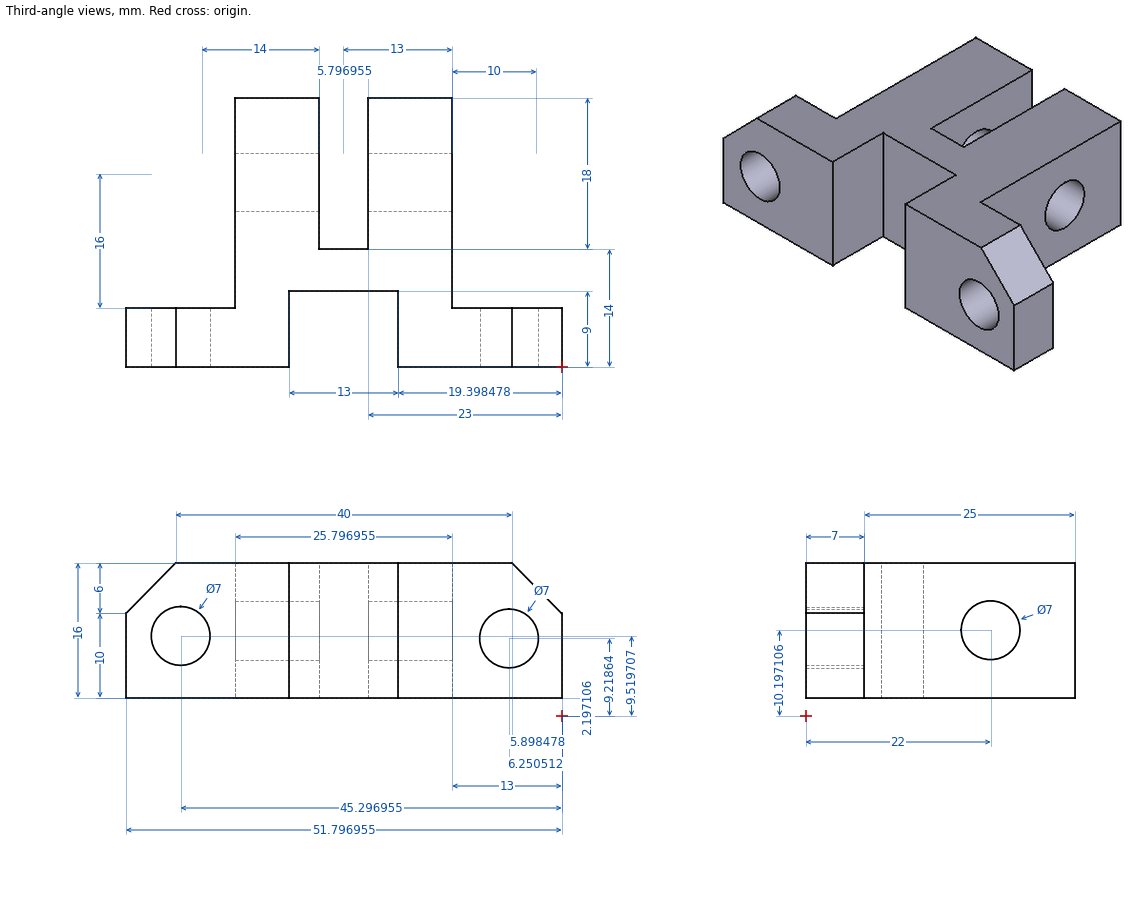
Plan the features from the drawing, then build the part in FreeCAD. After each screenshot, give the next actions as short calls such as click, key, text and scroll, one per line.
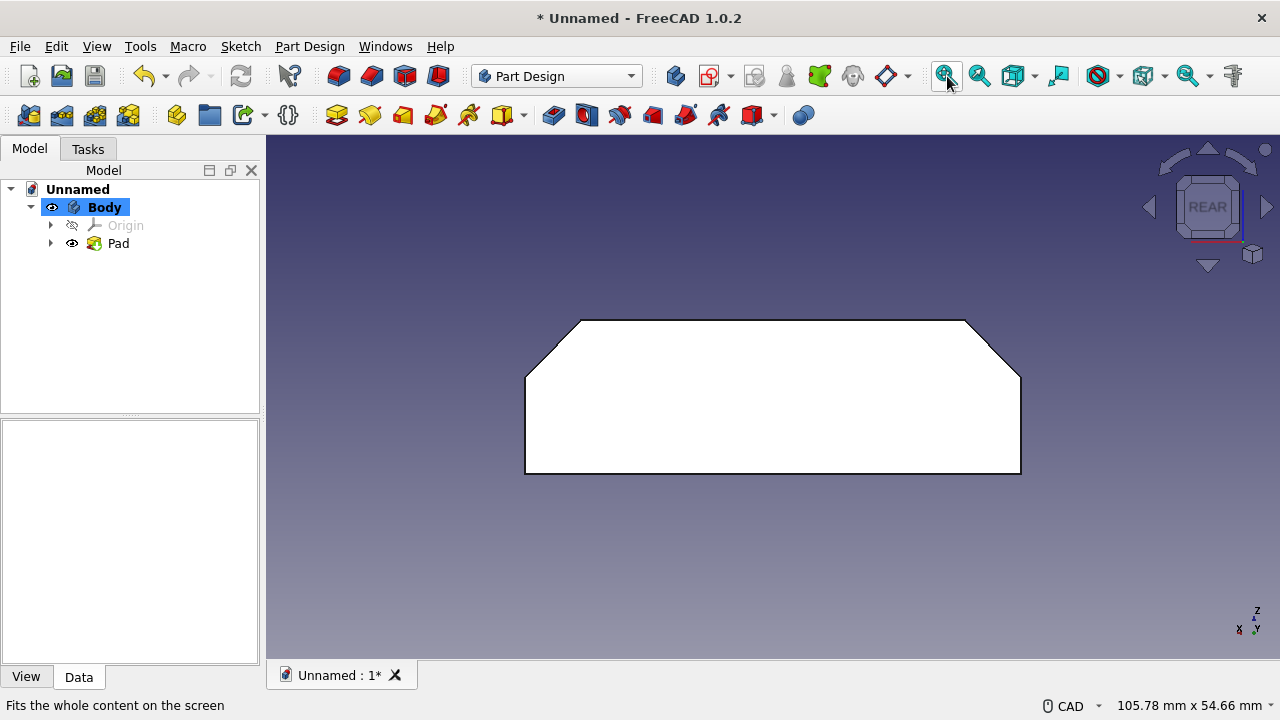
click(631, 396)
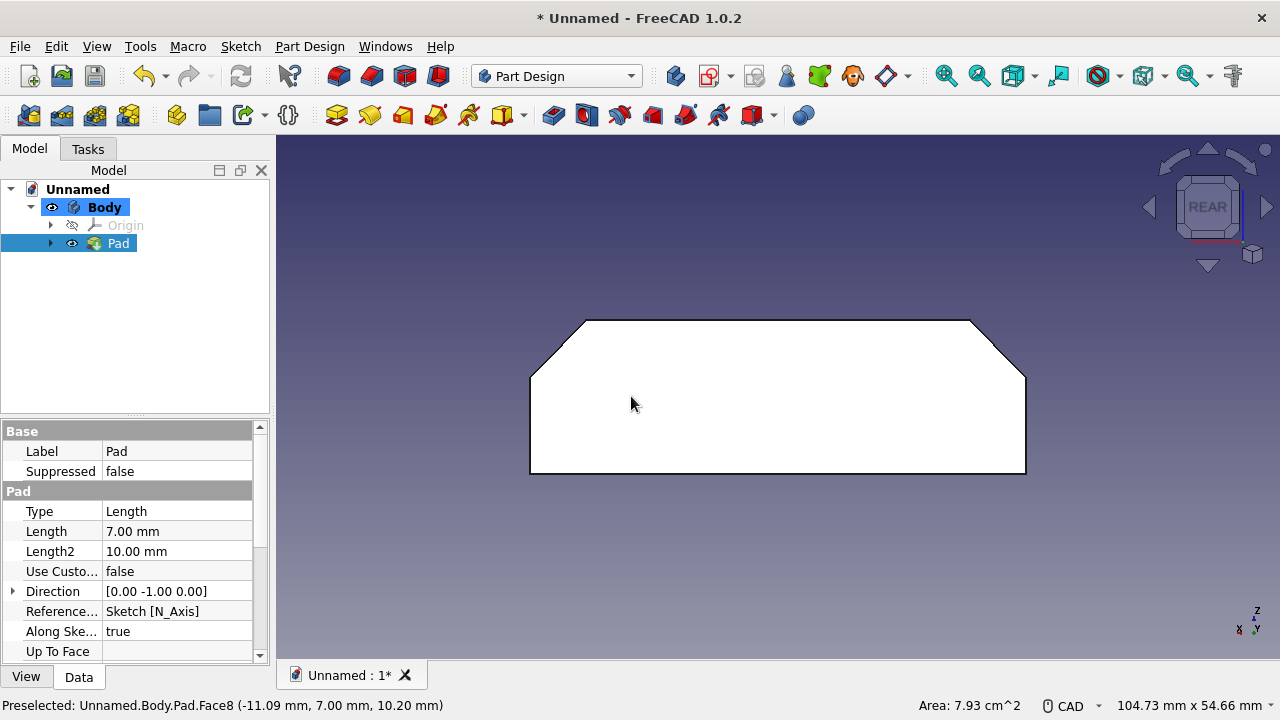
click(708, 76)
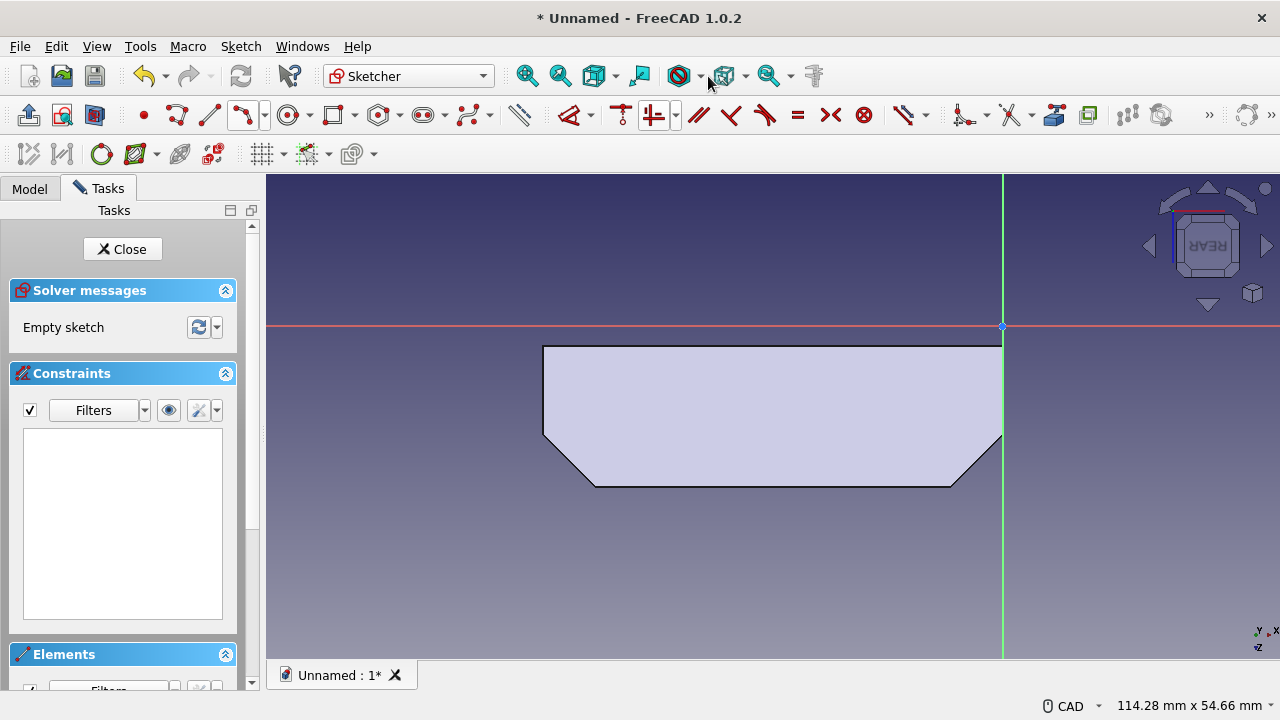
scroll(575, 409, up, 8)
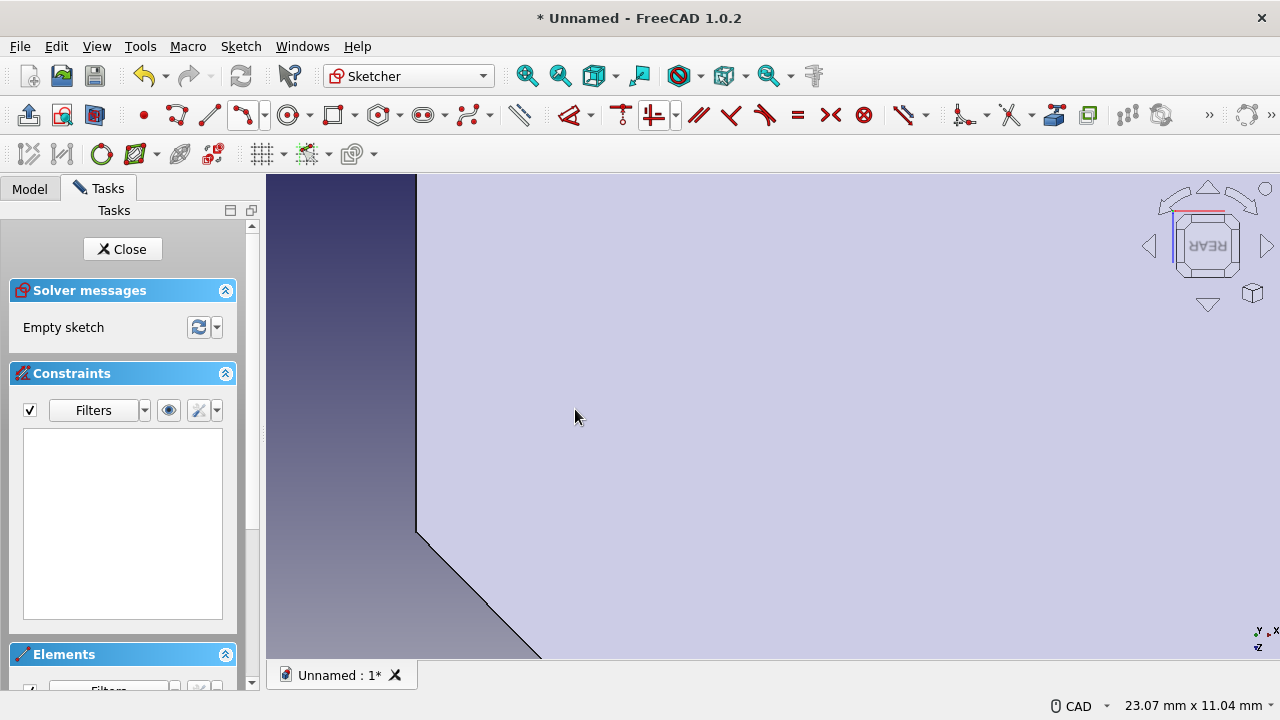
key(g)
key(c)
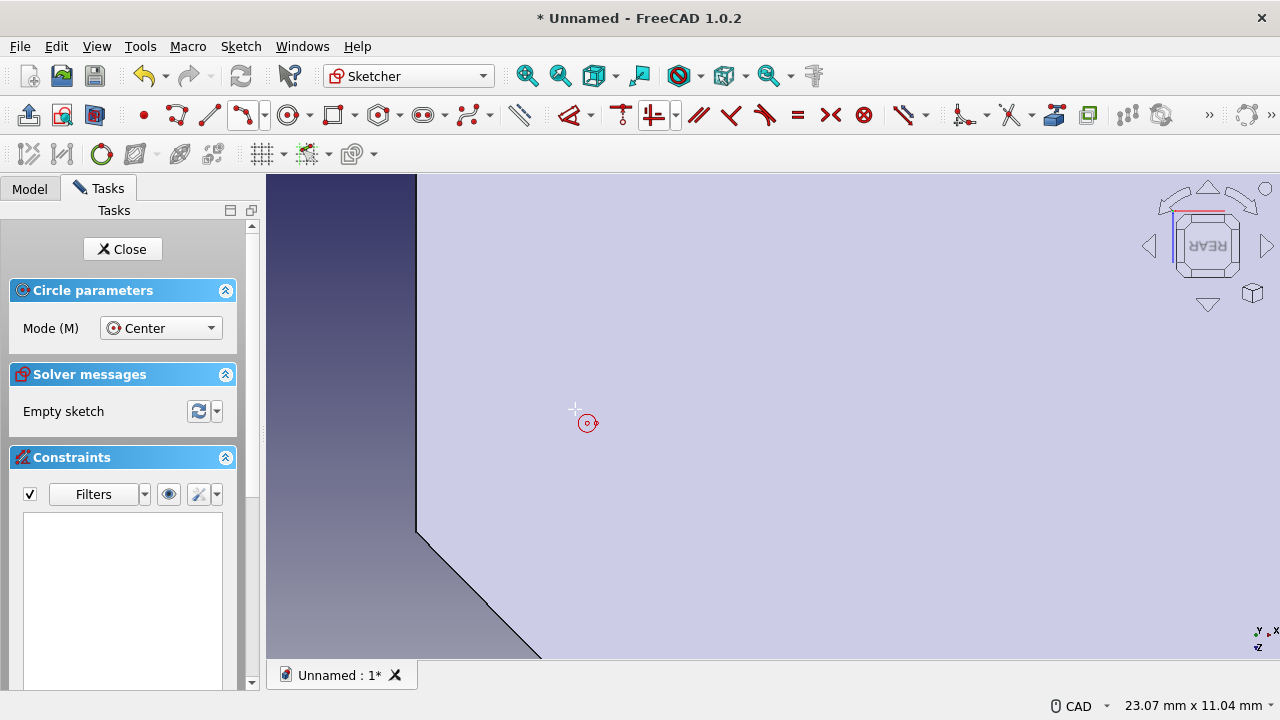
click(702, 414)
click(811, 306)
key(Escape)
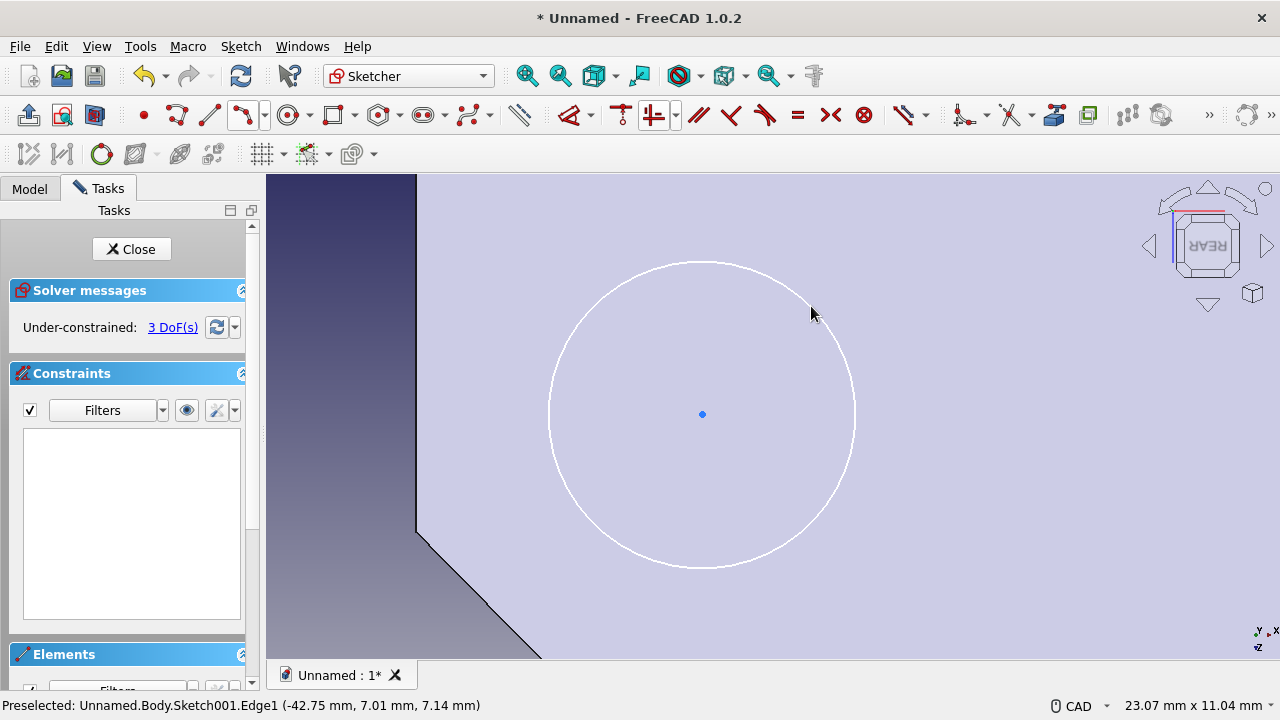
key(d)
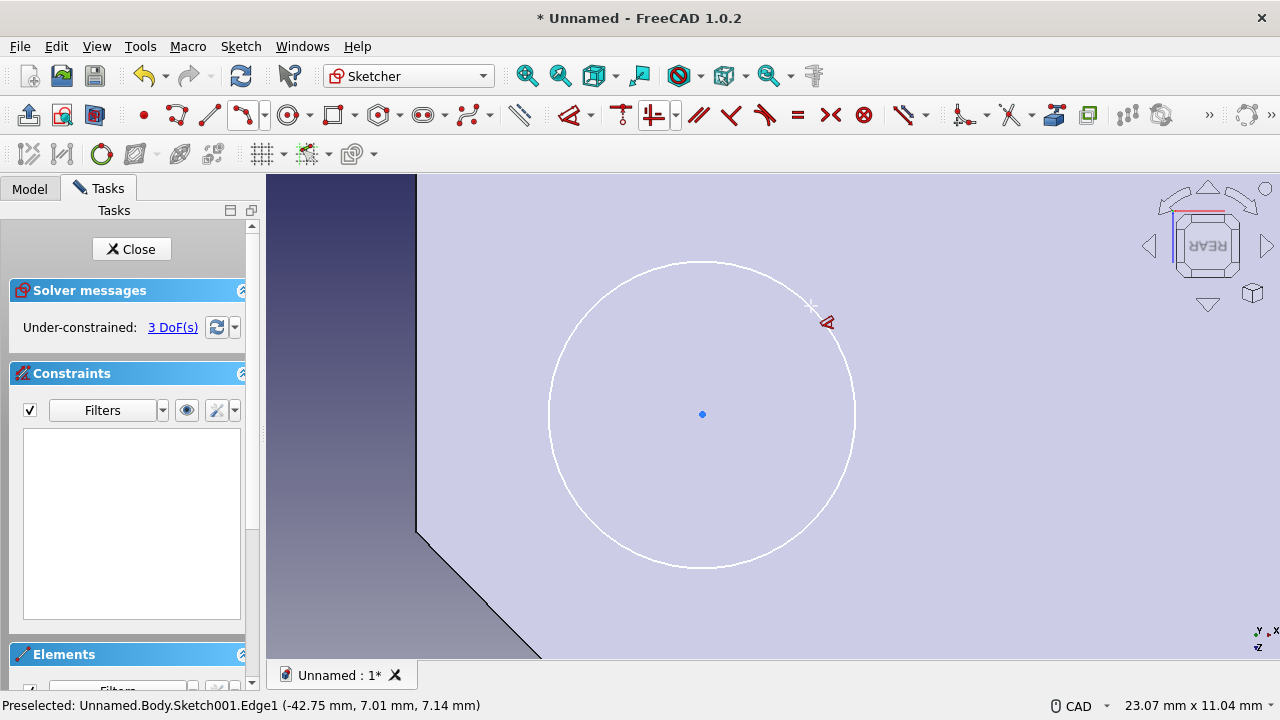
click(810, 306)
click(833, 283)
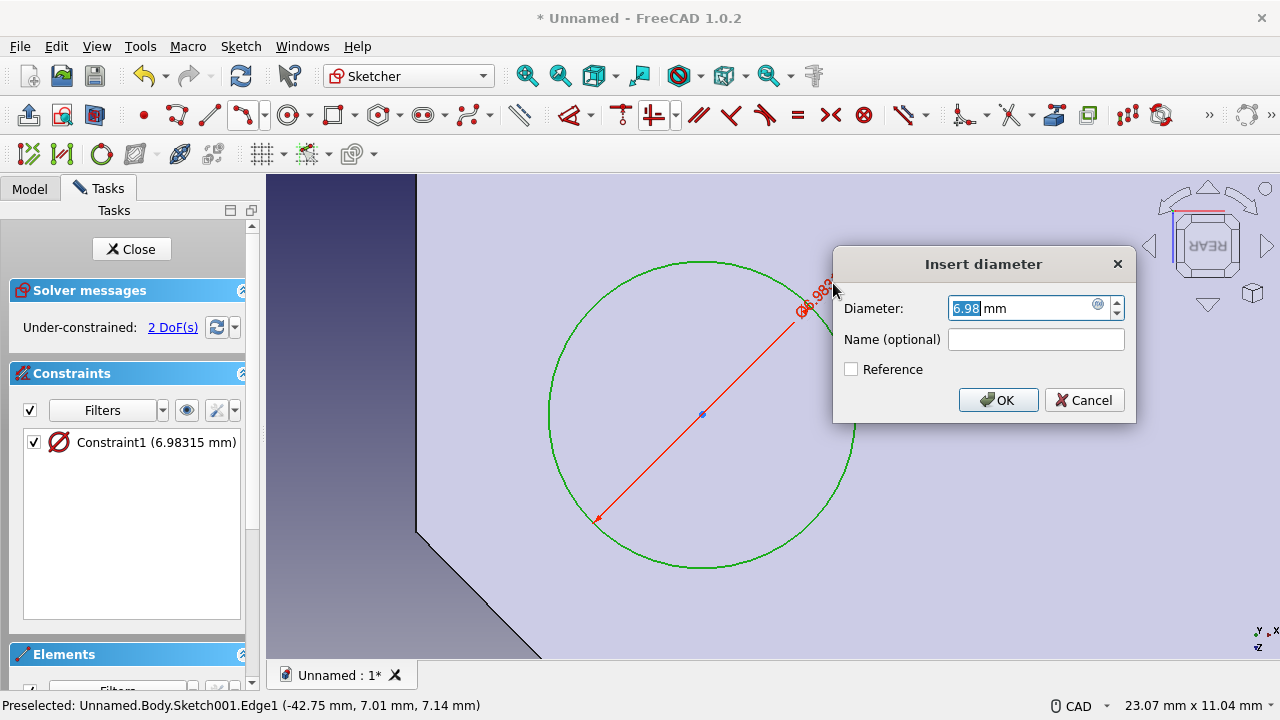
text(7)
key(Return)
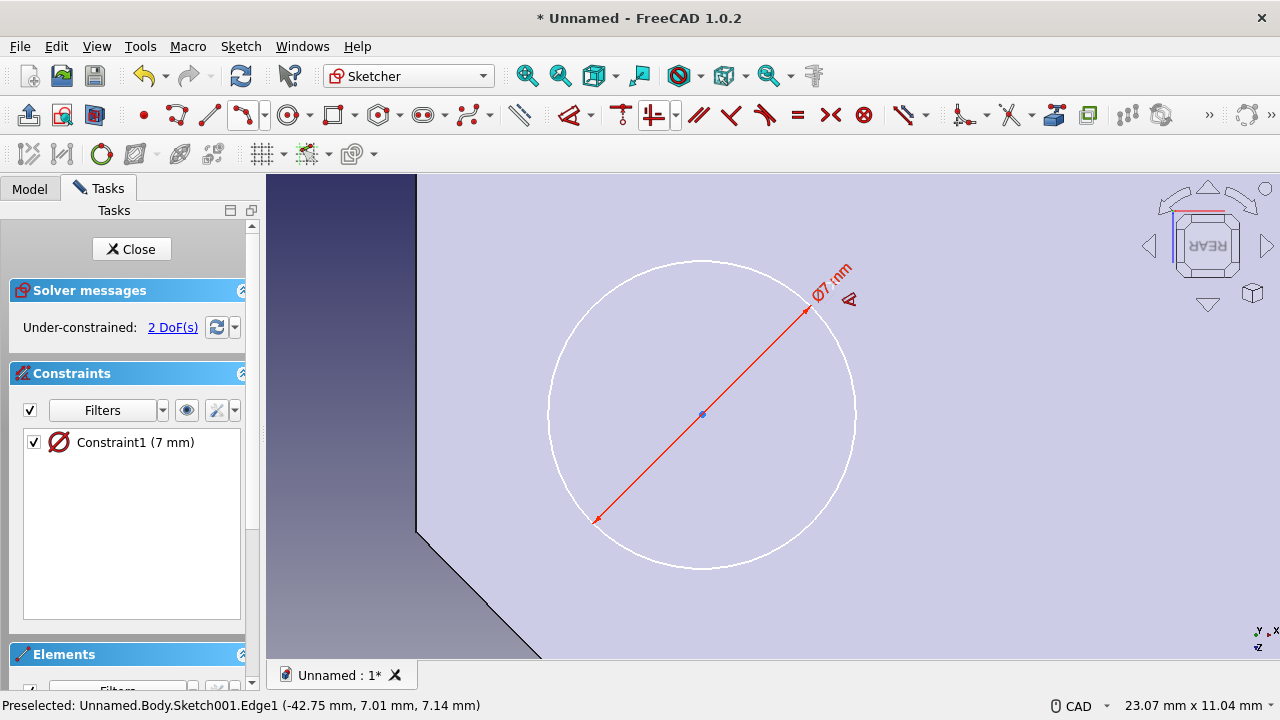
click(702, 415)
click(668, 308)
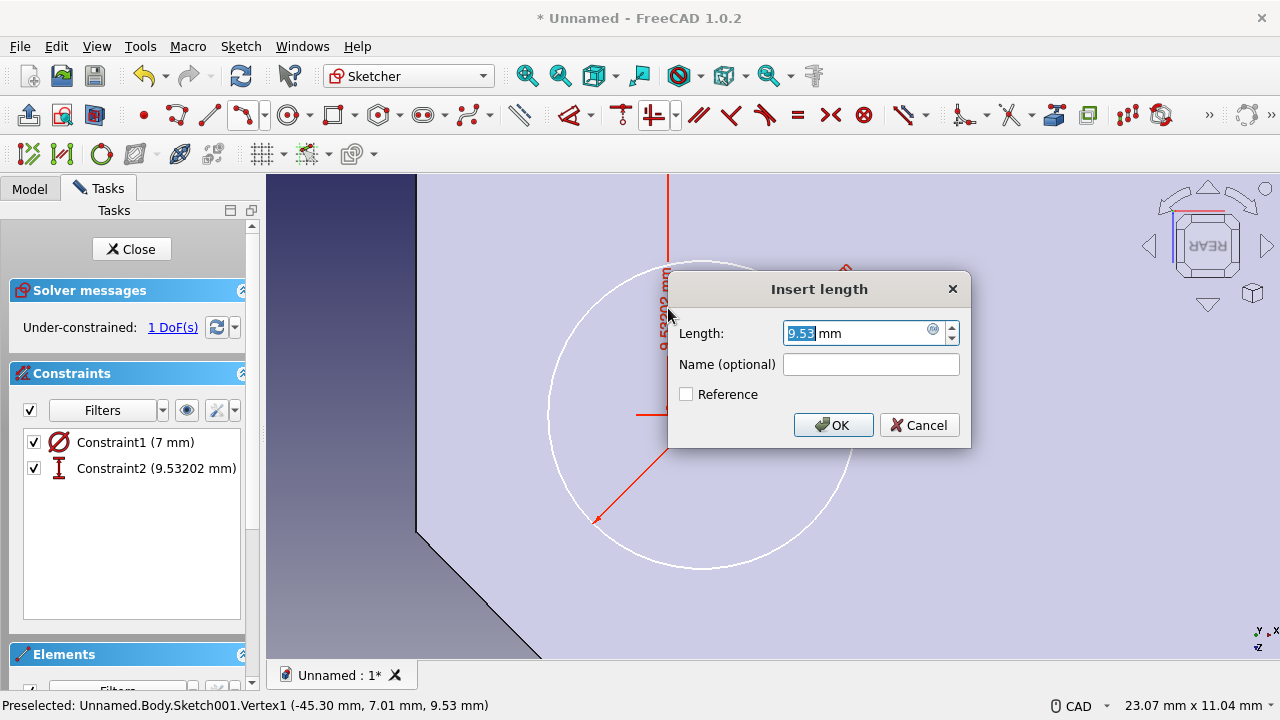
text(9.519707)
key(Return)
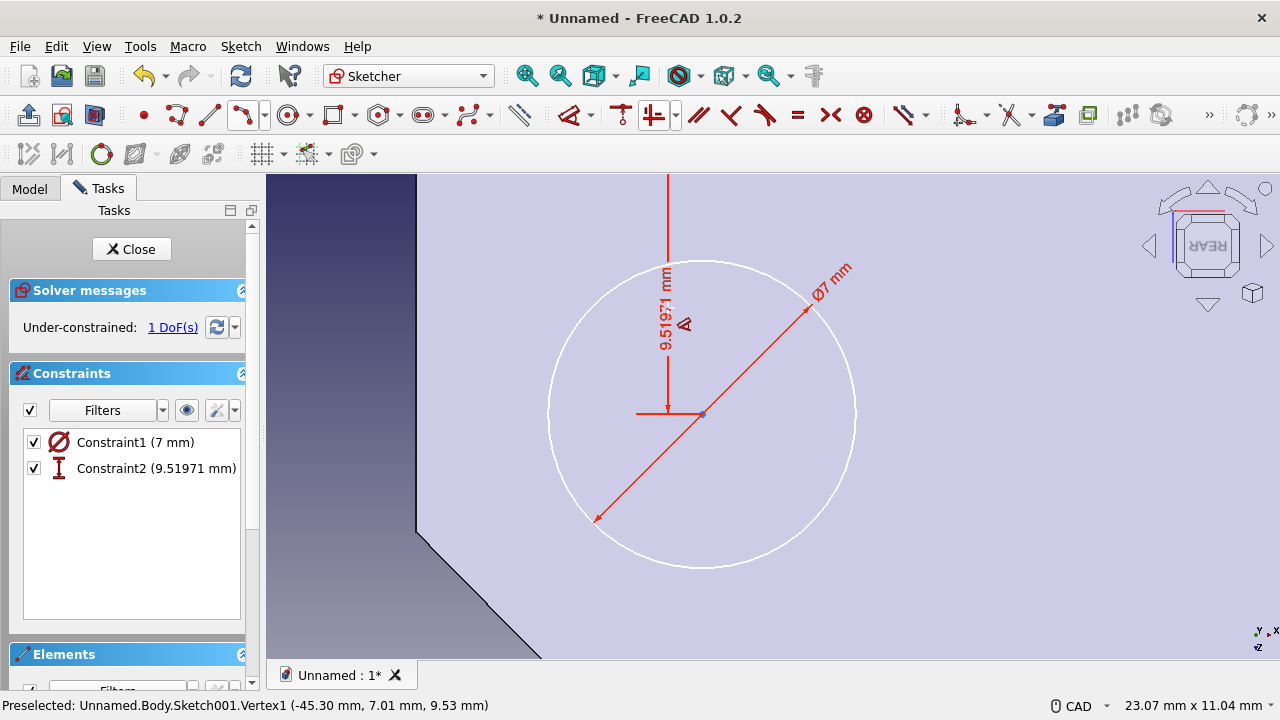
click(702, 414)
click(909, 448)